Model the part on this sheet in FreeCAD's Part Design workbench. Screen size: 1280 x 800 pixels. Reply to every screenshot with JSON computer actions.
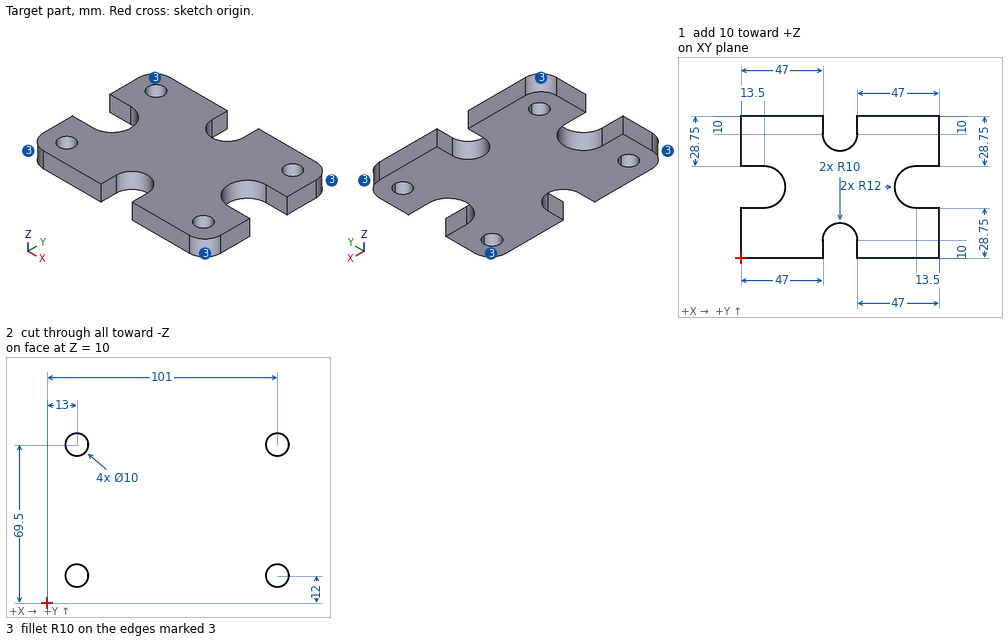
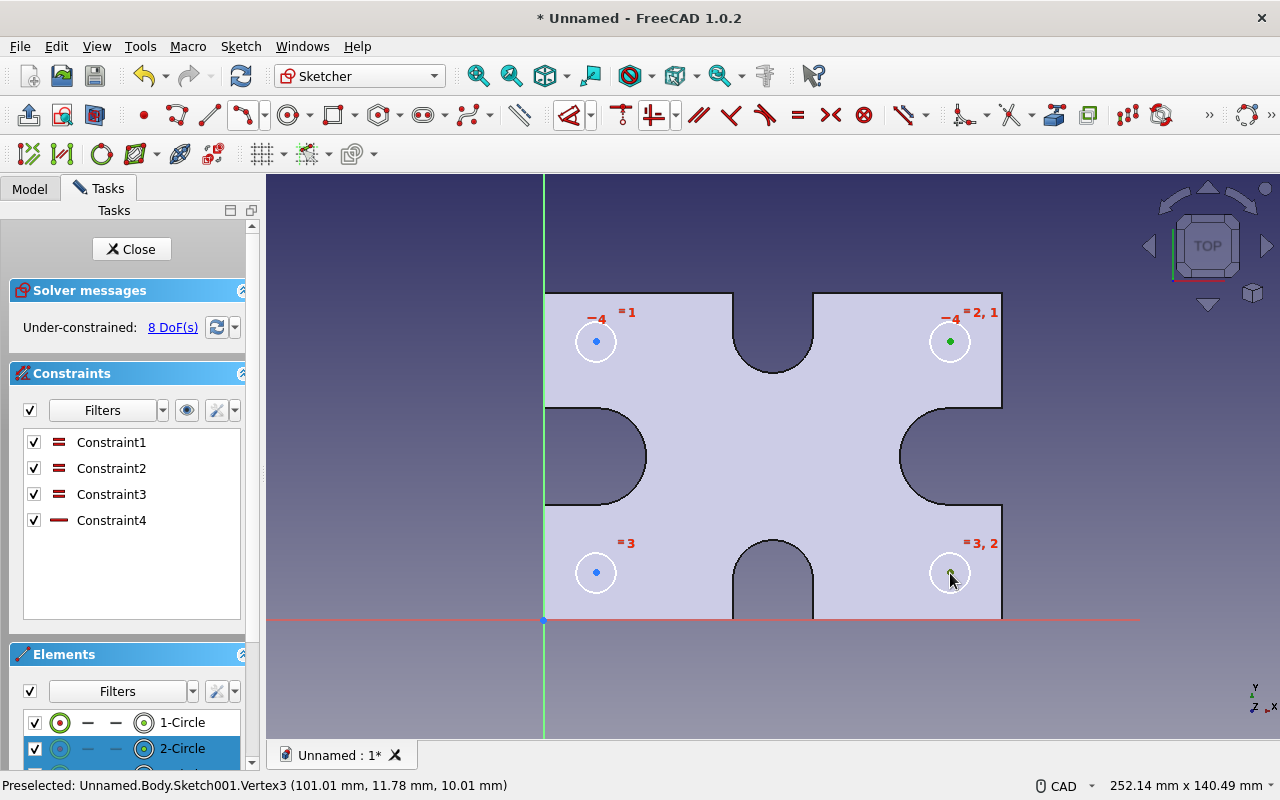
{"action": "left_click", "coordinate": [676, 116]}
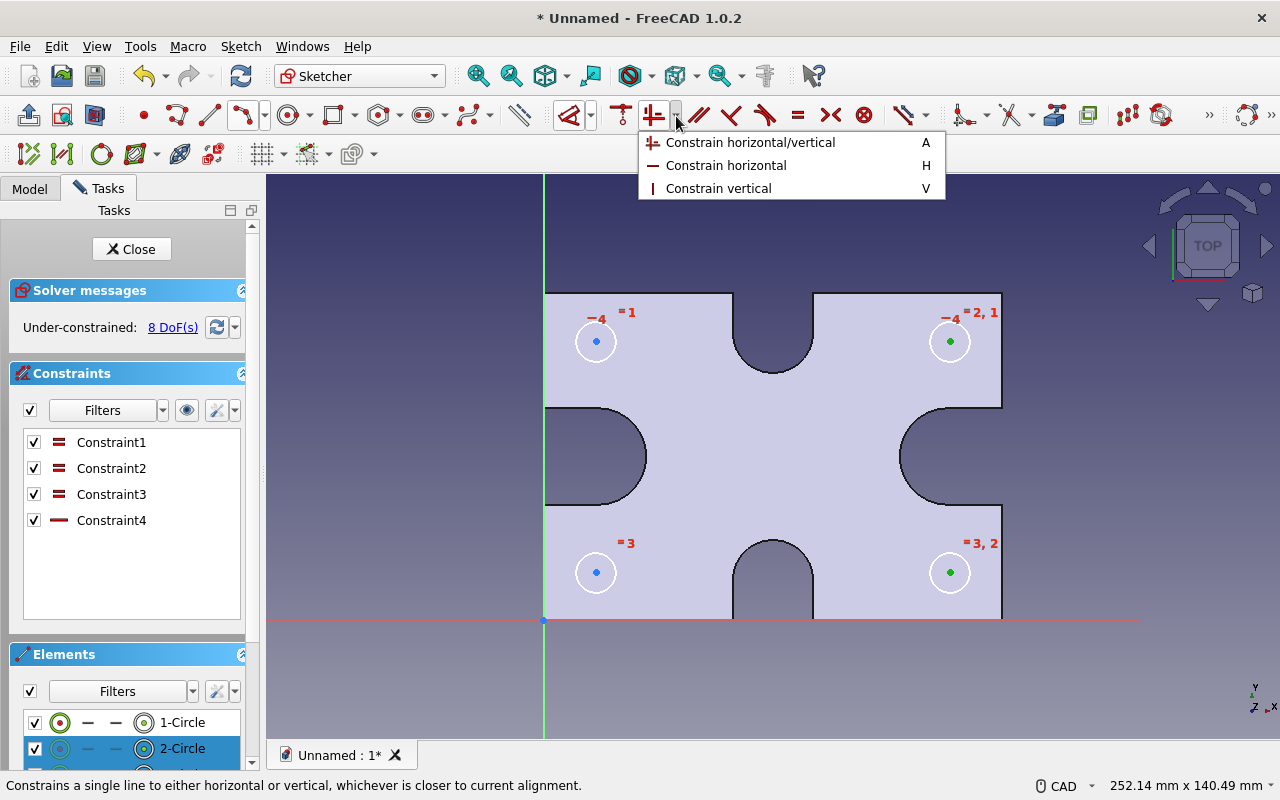
{"action": "left_click", "coordinate": [792, 188]}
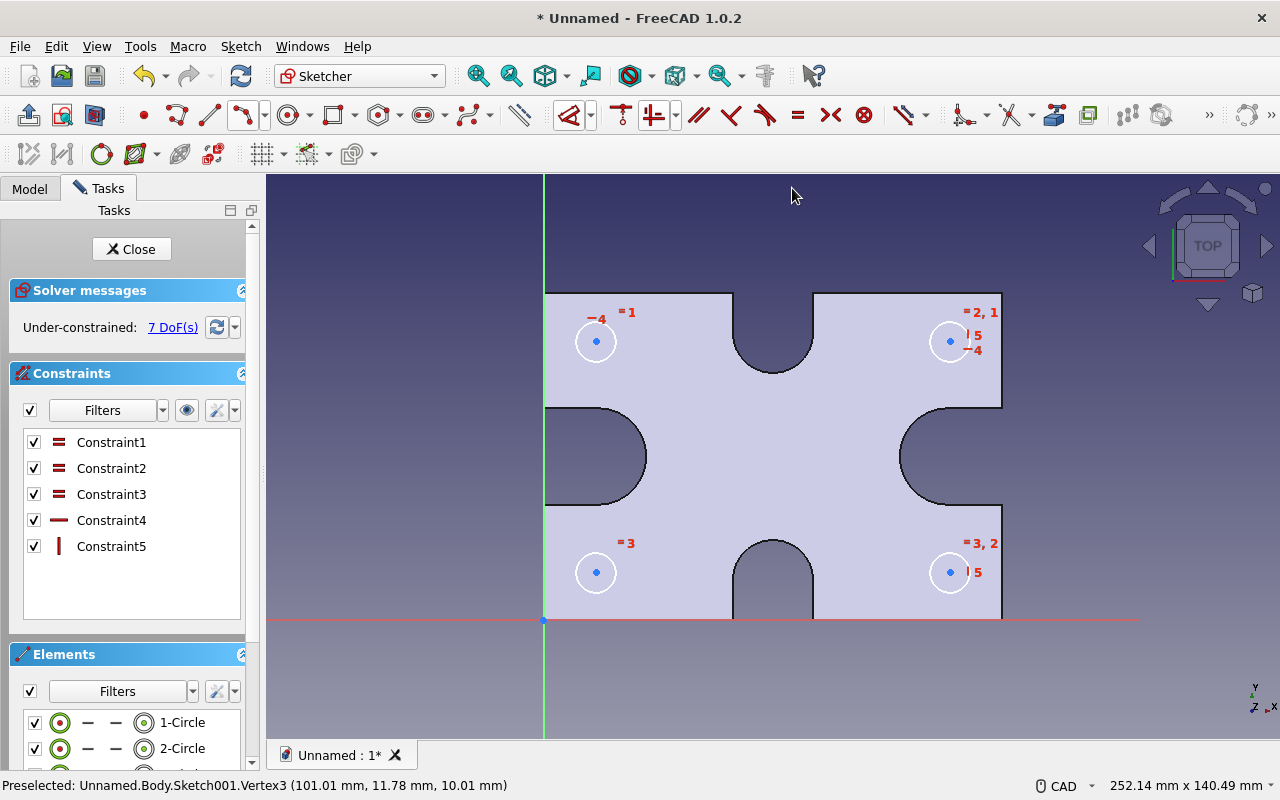
{"action": "left_click", "coordinate": [596, 342]}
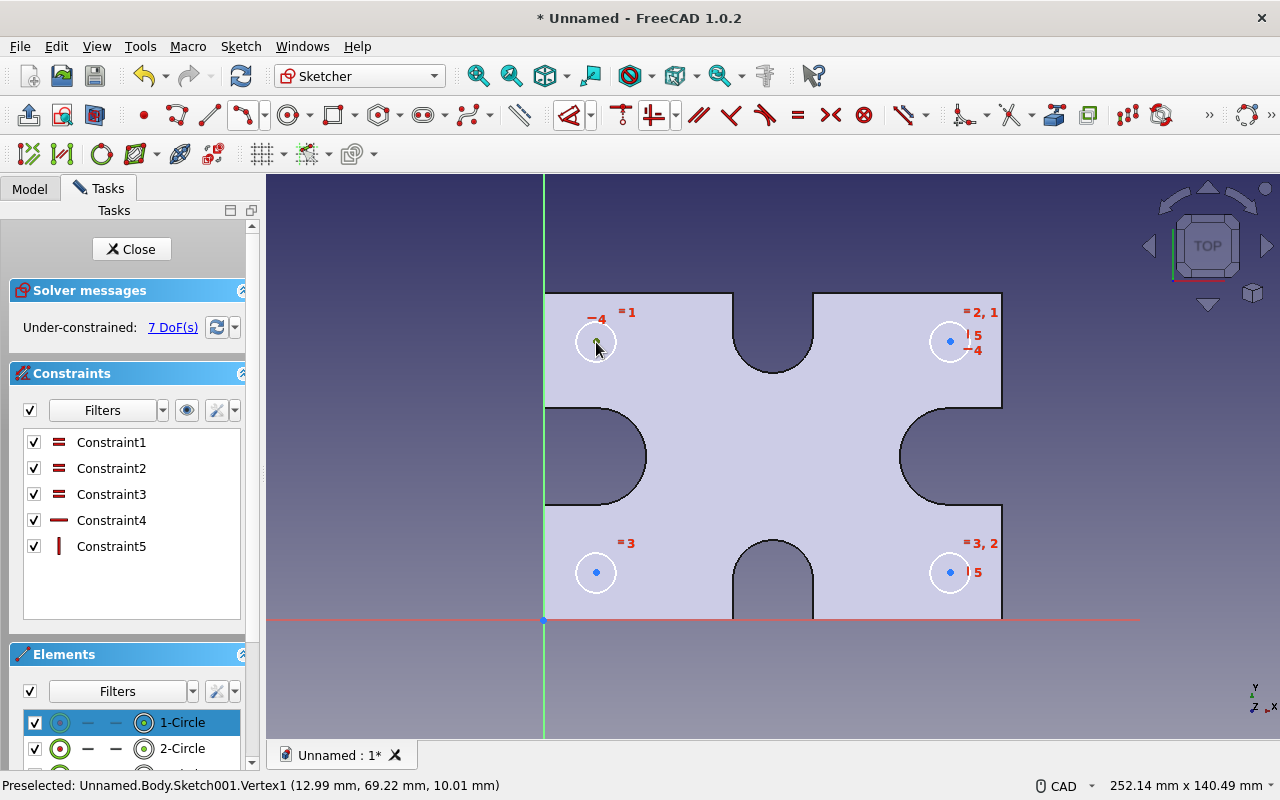
{"action": "left_click", "coordinate": [596, 573]}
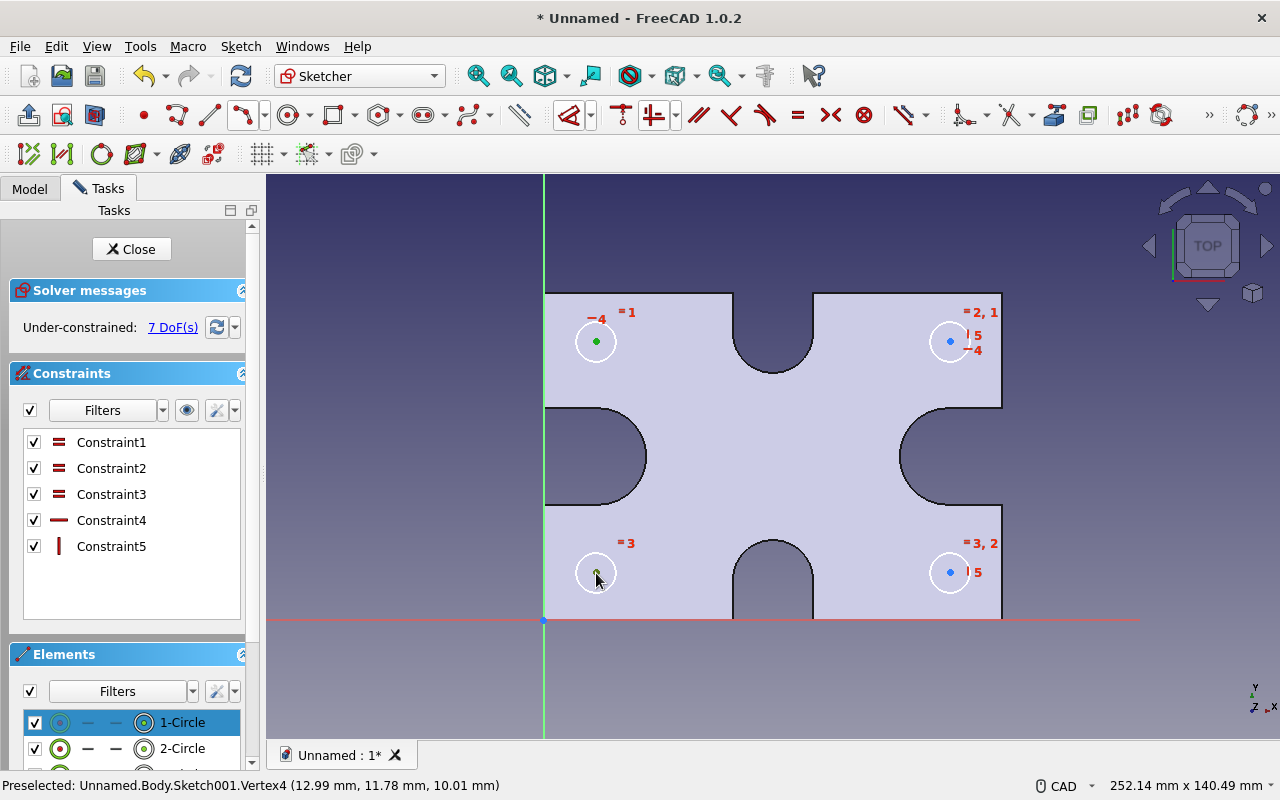
{"action": "key", "text": "v"}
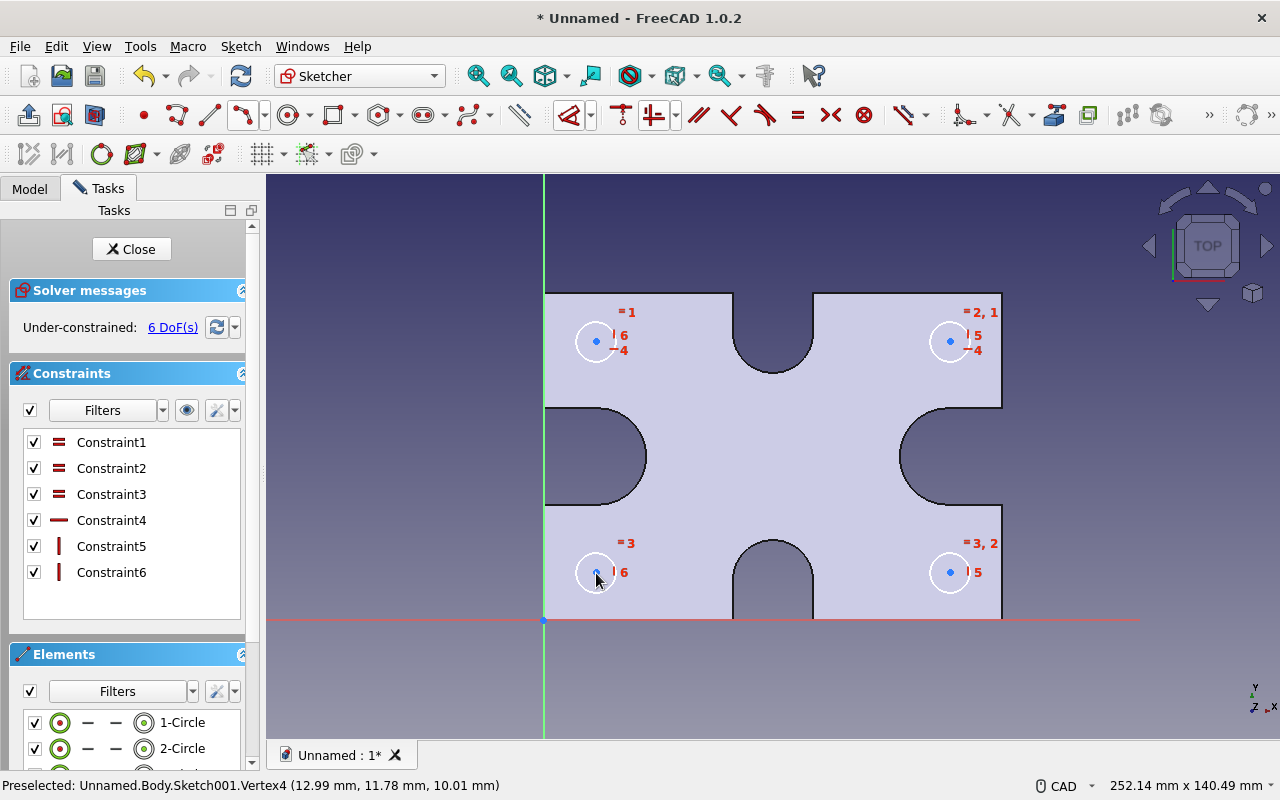
{"action": "left_click", "coordinate": [950, 573]}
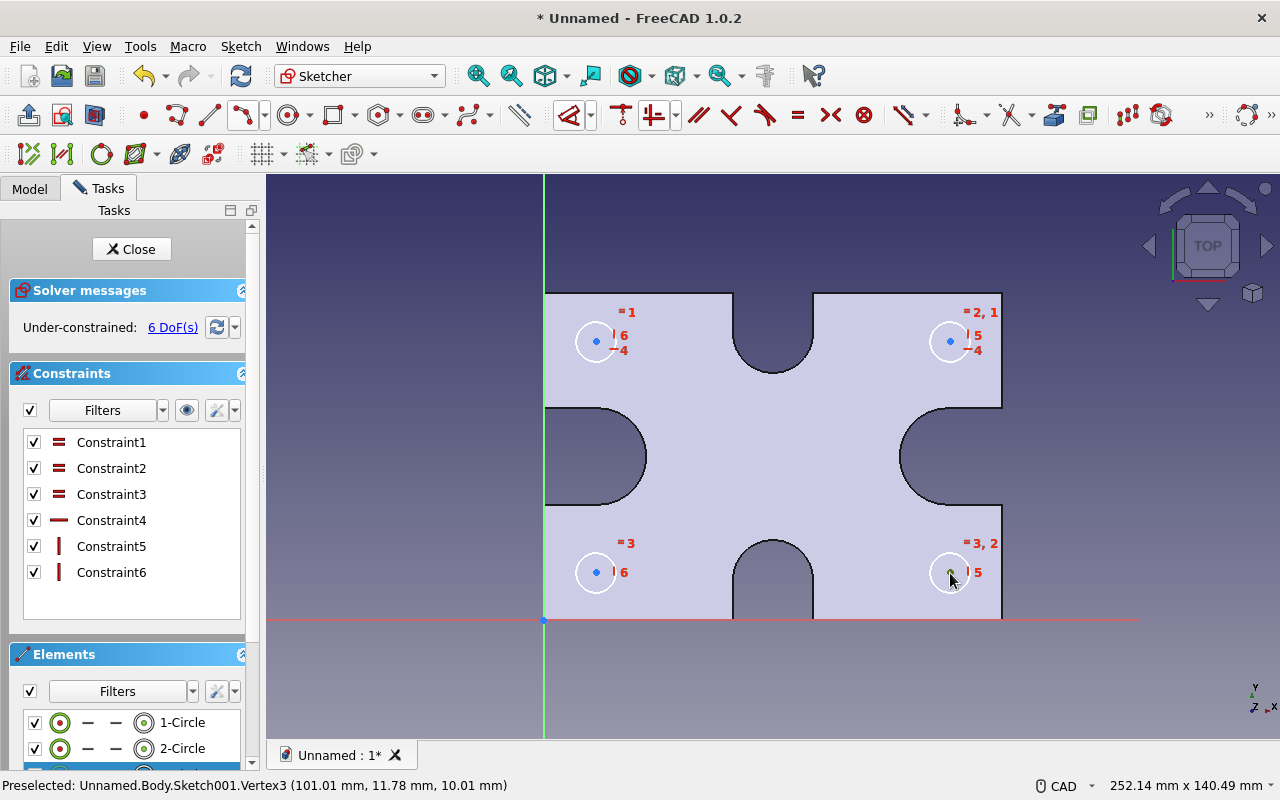
{"action": "left_click", "coordinate": [596, 573]}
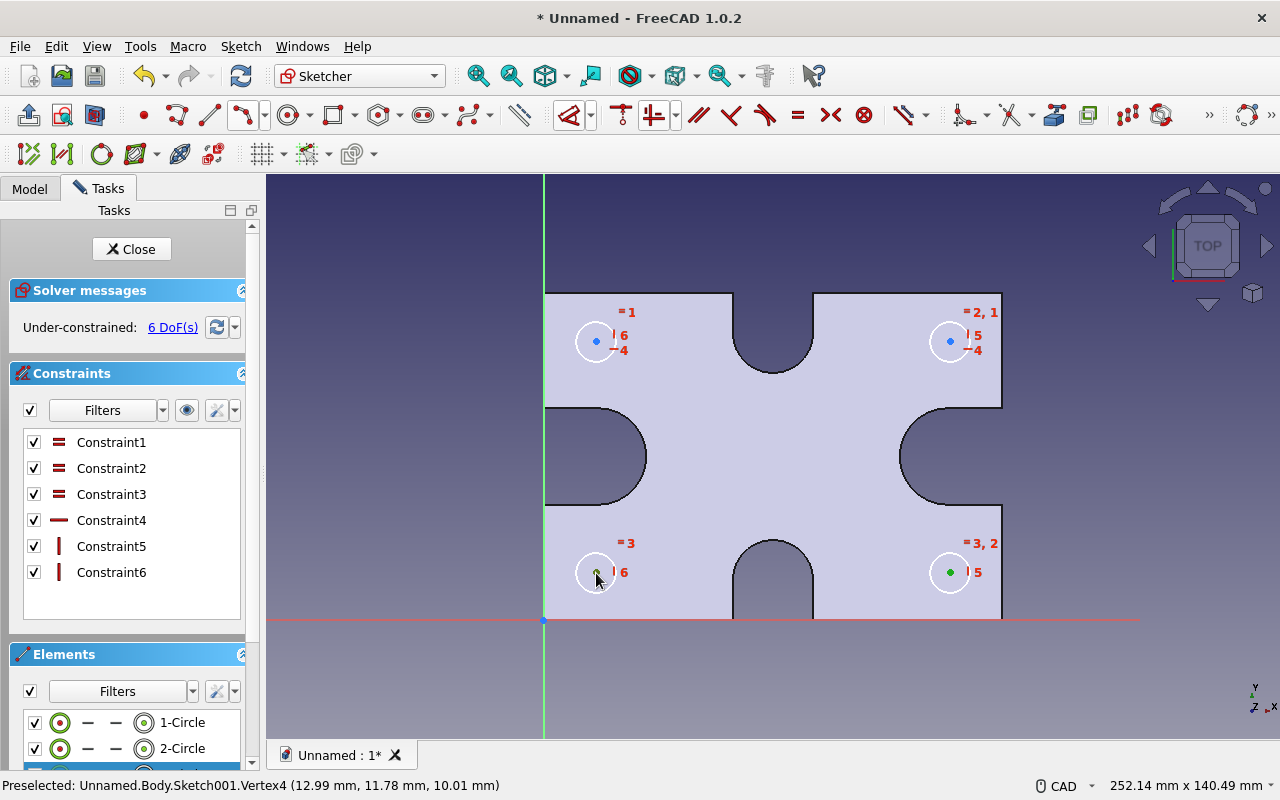
{"action": "left_click", "coordinate": [676, 116]}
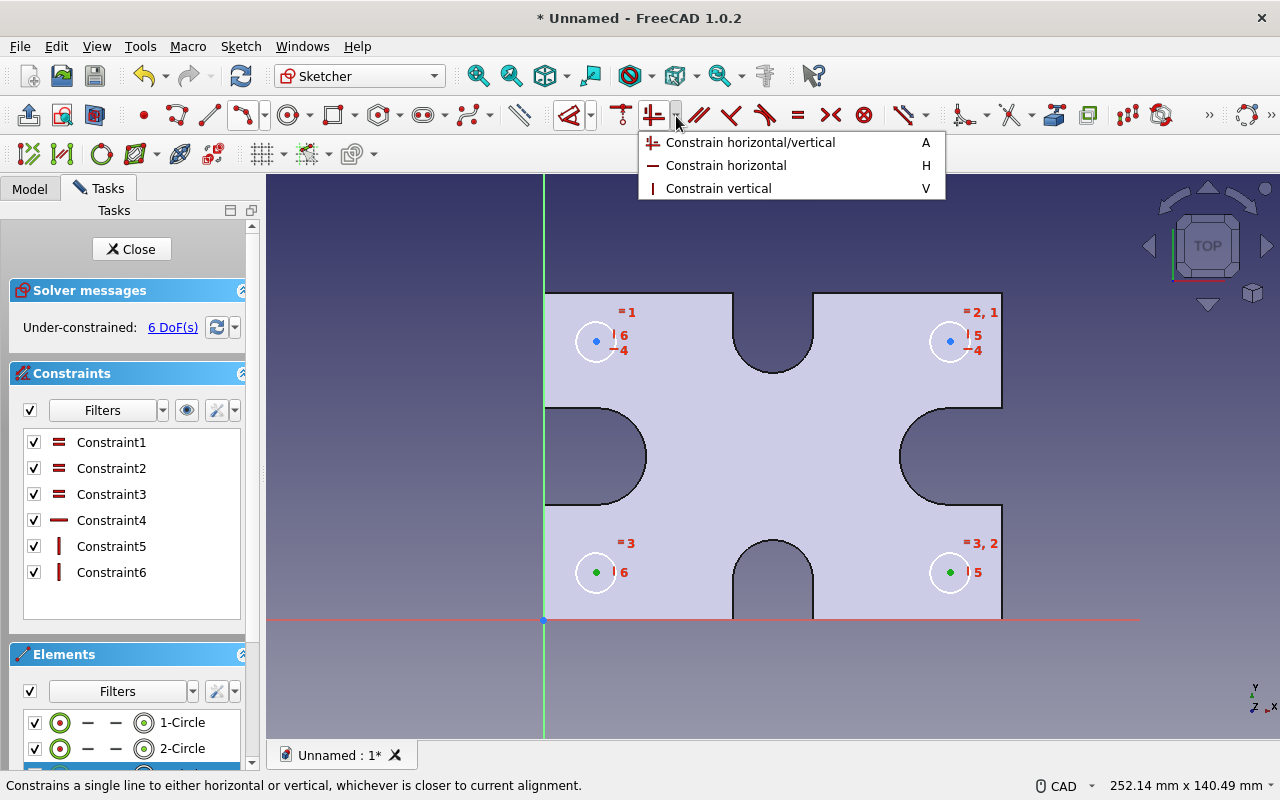
{"action": "left_click", "coordinate": [792, 166]}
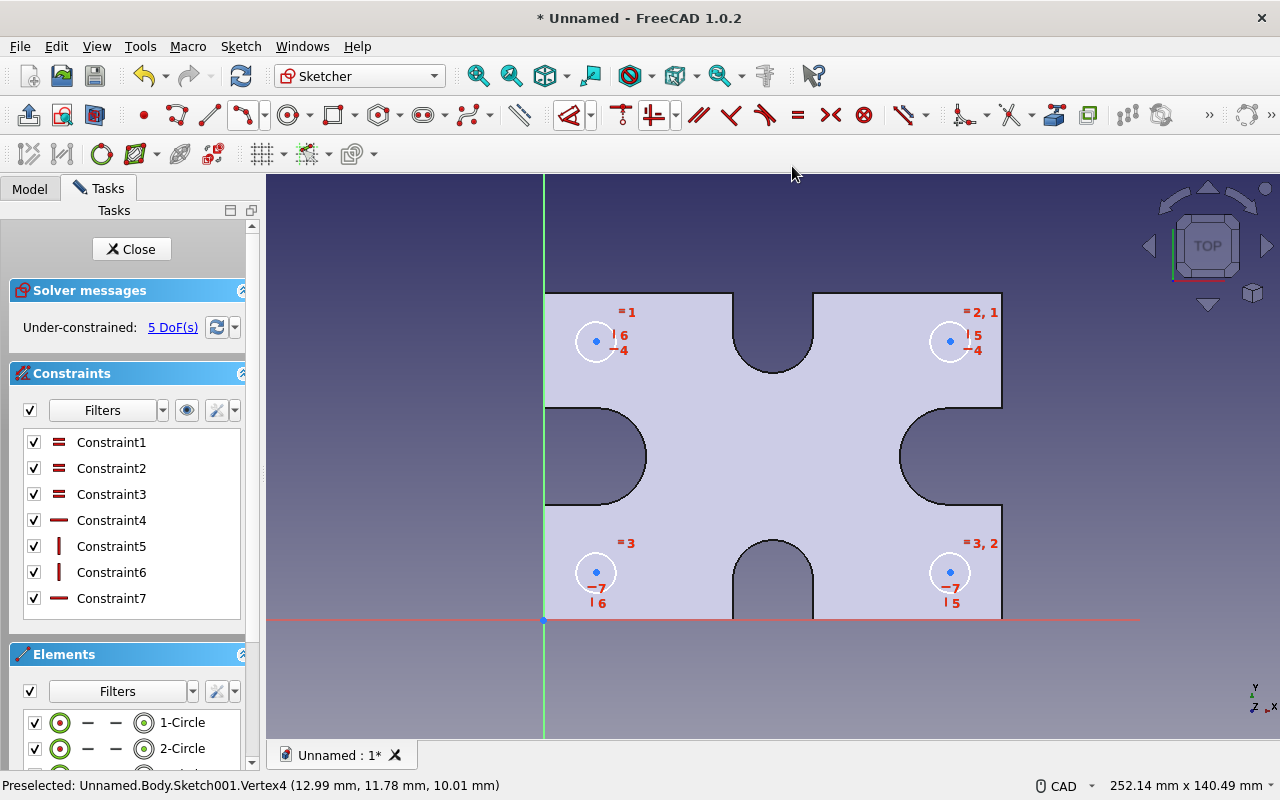
{"action": "left_click", "coordinate": [582, 328]}